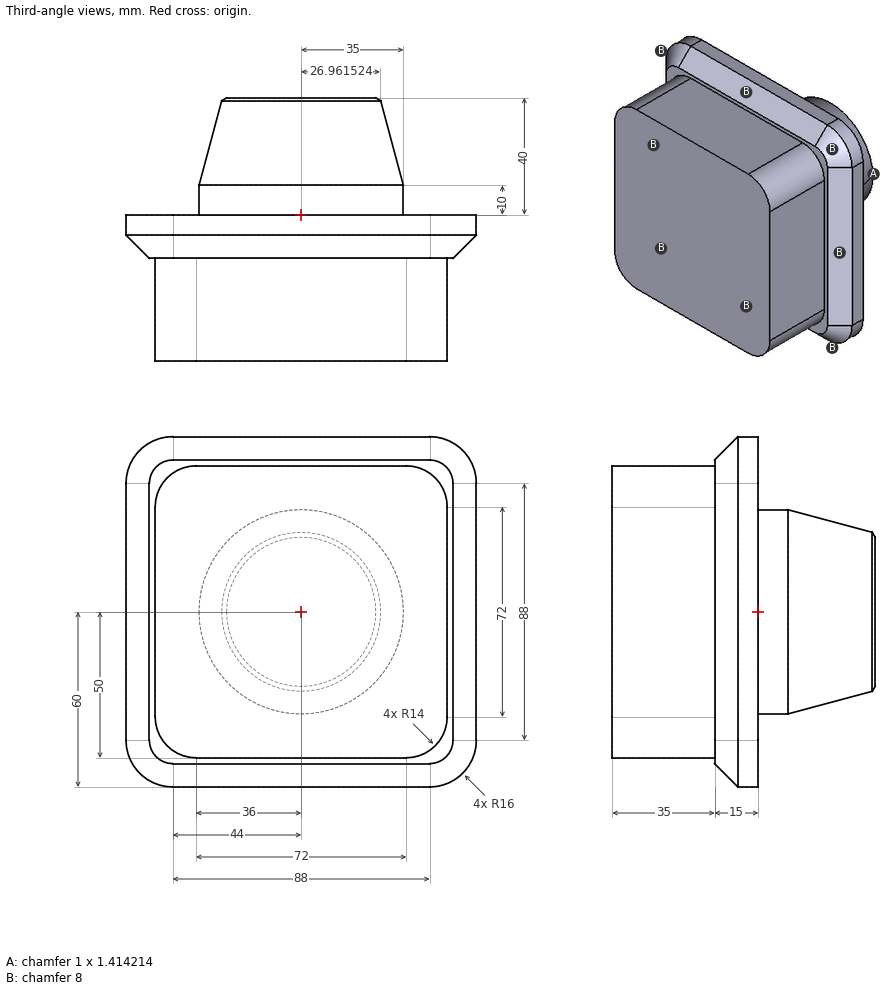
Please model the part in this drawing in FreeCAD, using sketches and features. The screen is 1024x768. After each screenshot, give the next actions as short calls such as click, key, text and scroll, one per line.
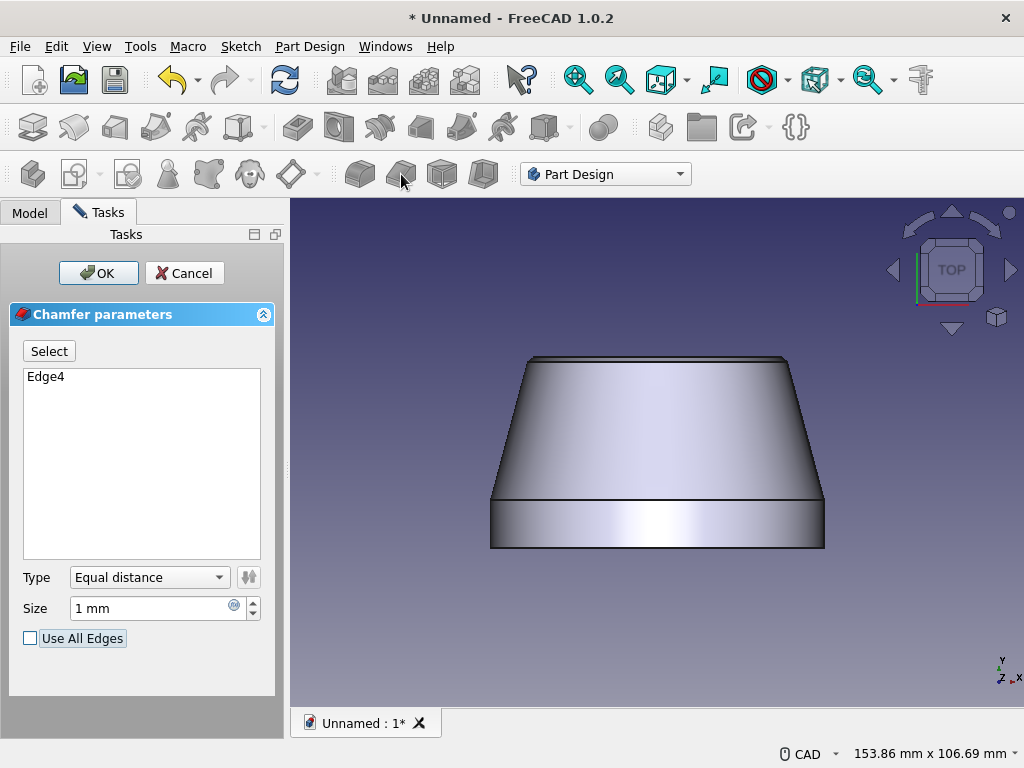
click(150, 578)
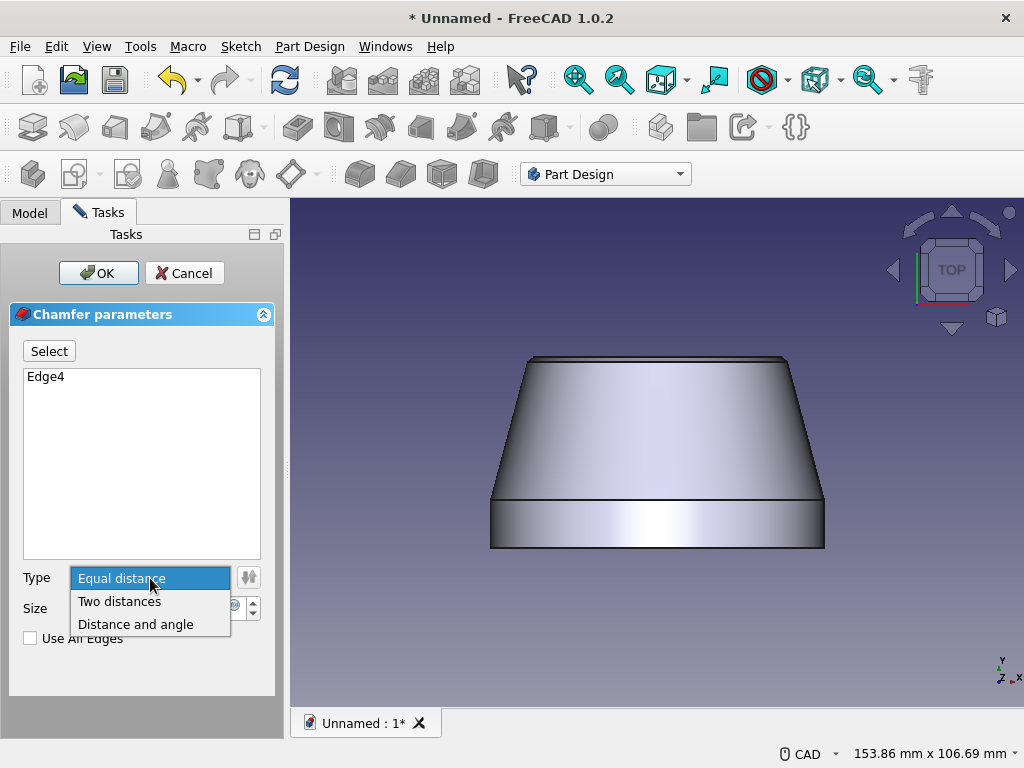
click(148, 602)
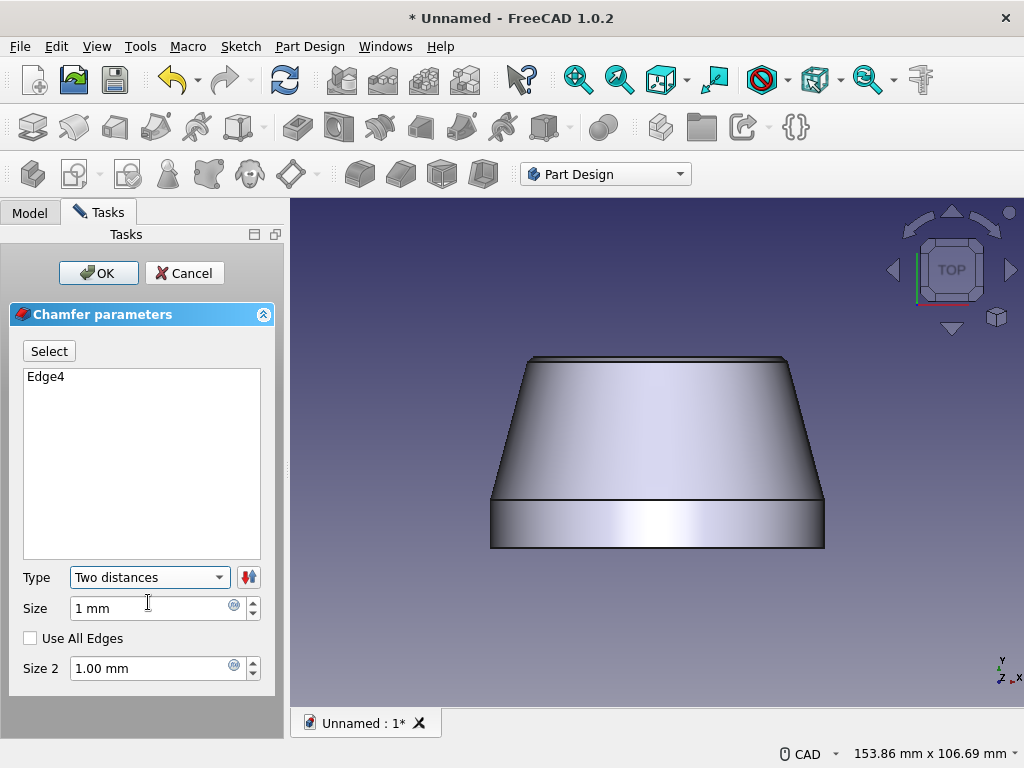
triple_click(158, 668)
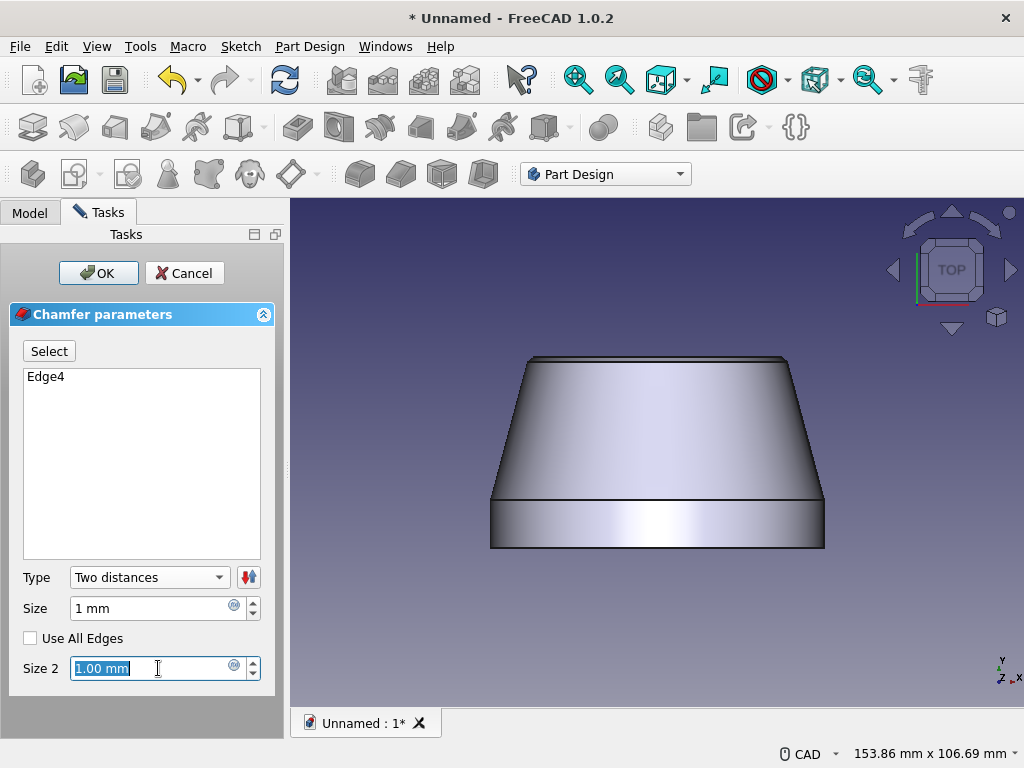
text(1.414214)
key(Tab)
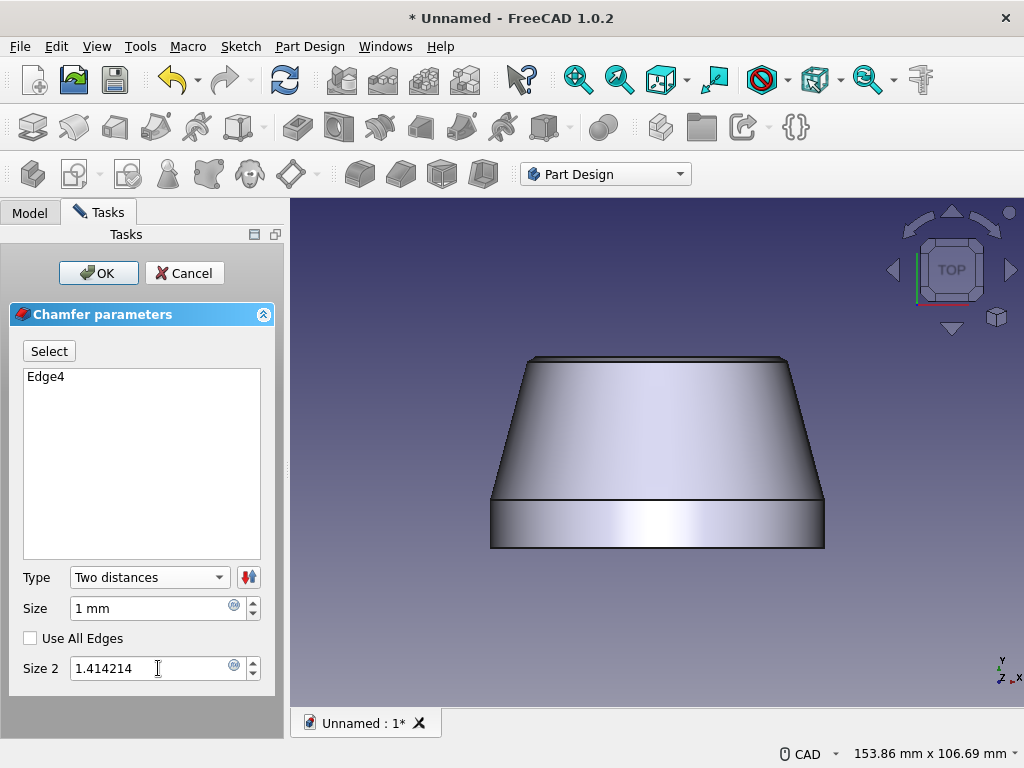
click(99, 273)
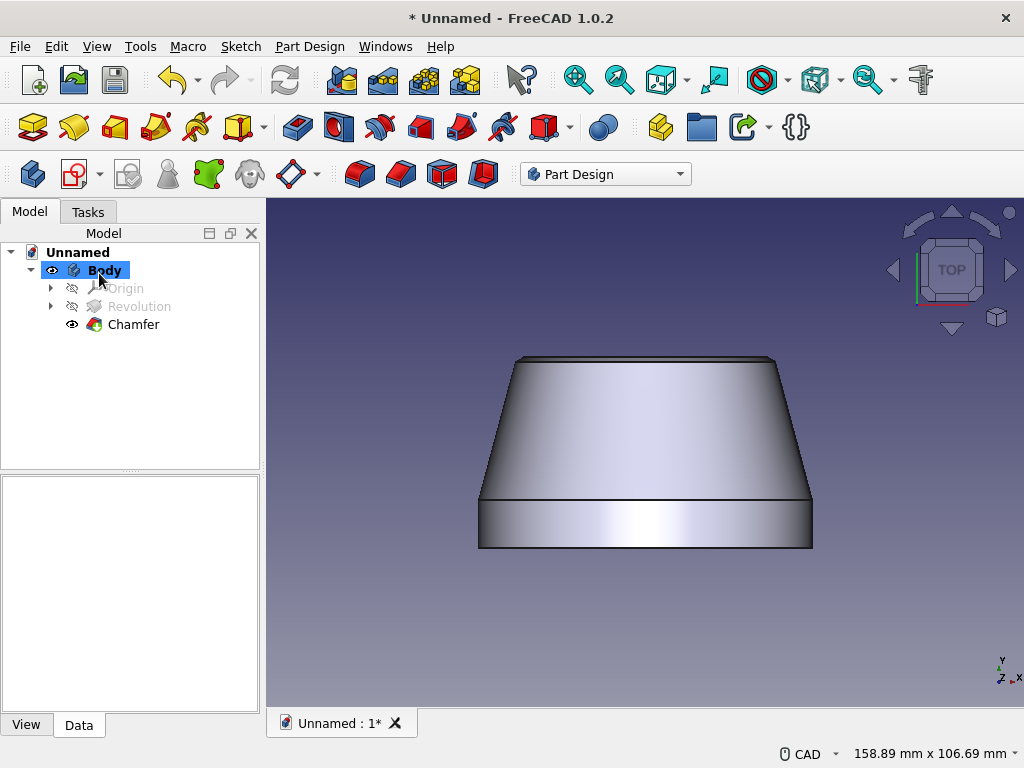
click(579, 80)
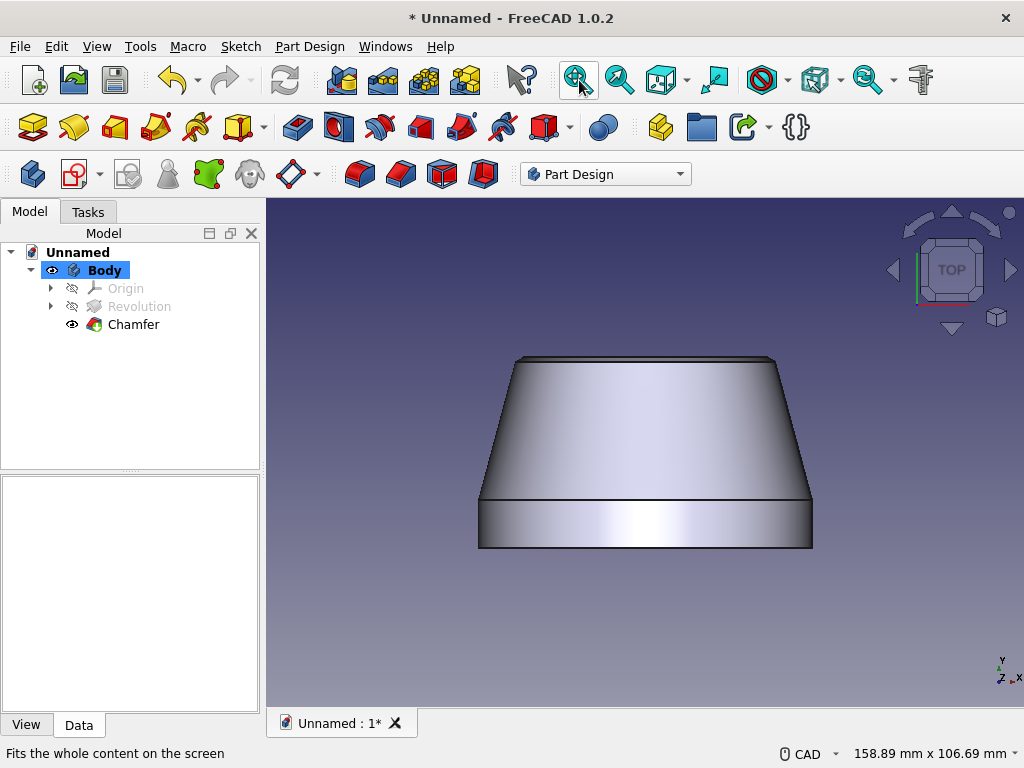
key(0)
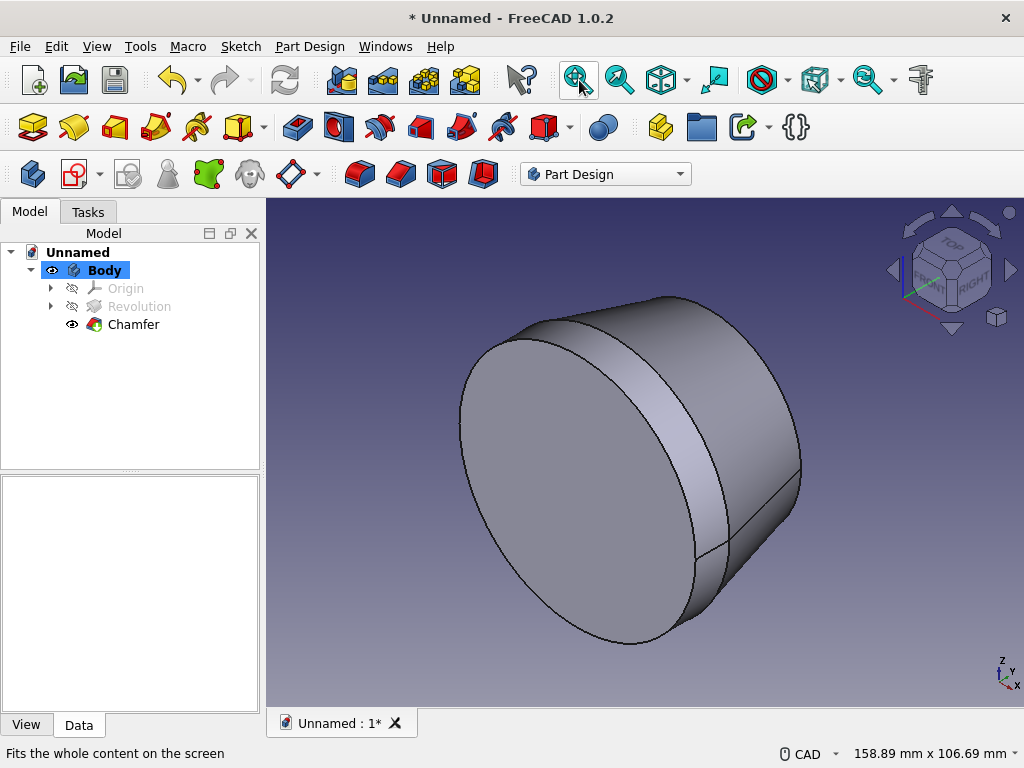
click(578, 490)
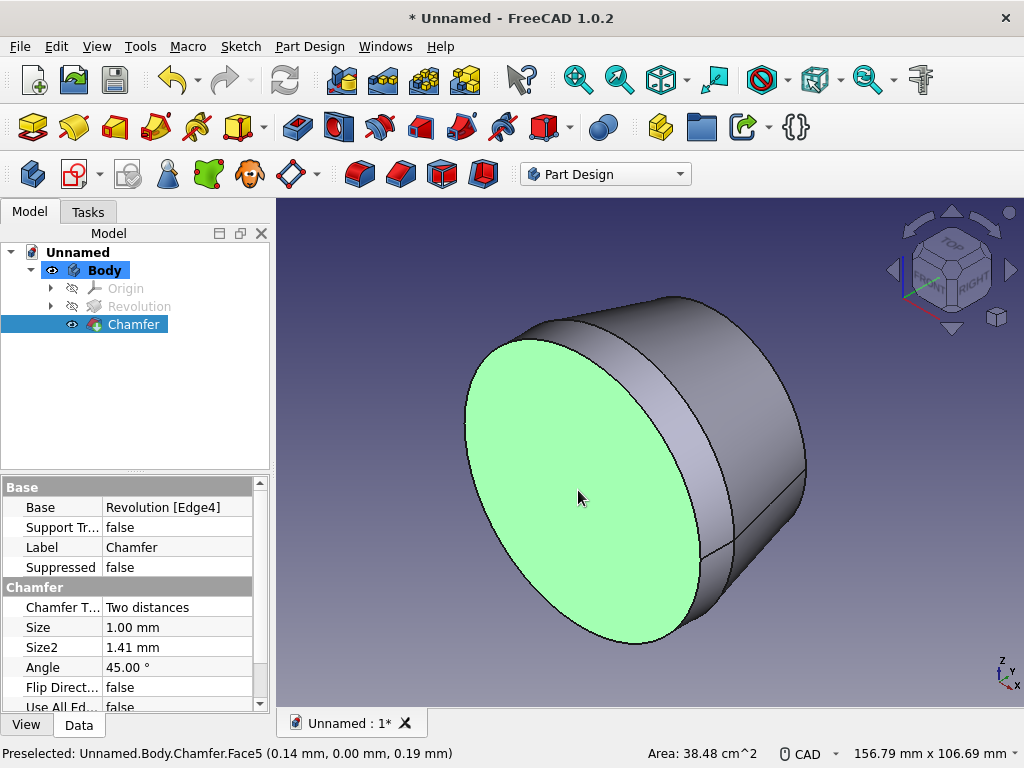
click(74, 174)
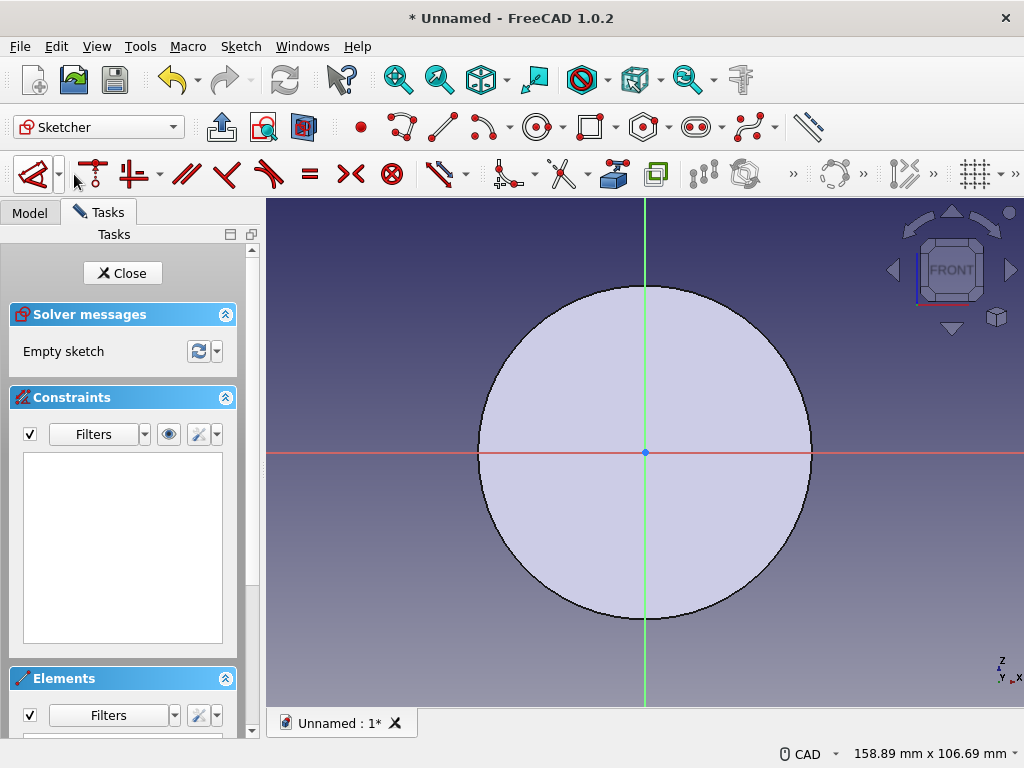
scroll(493, 452, down, 3)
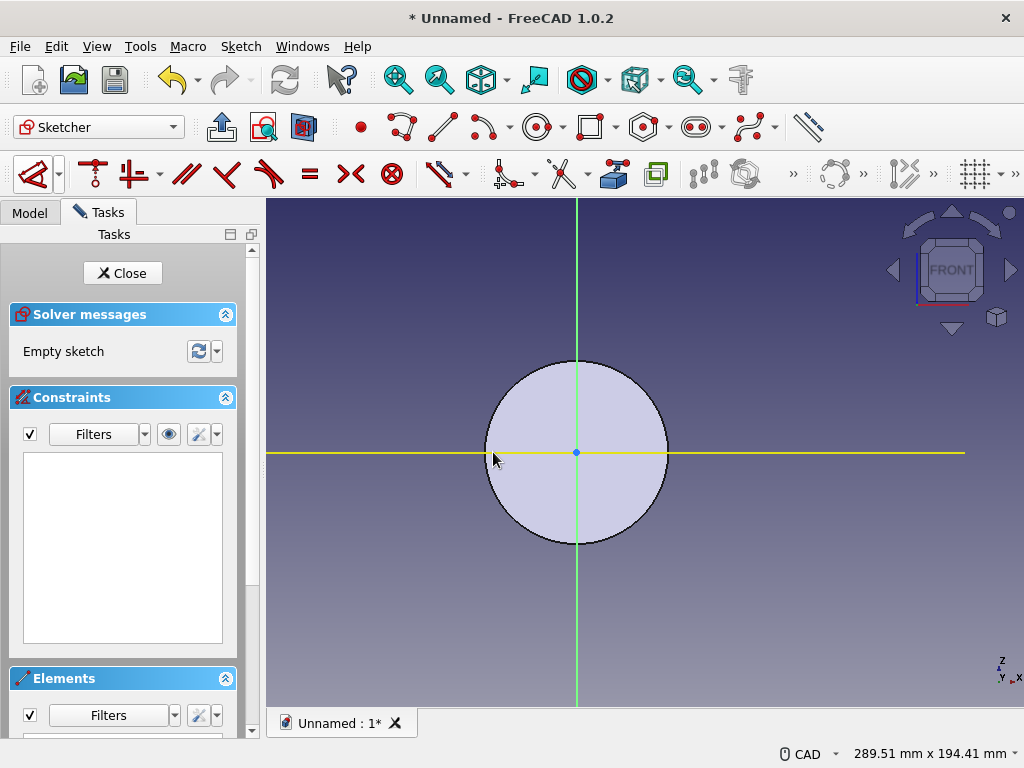
key(g)
key(l)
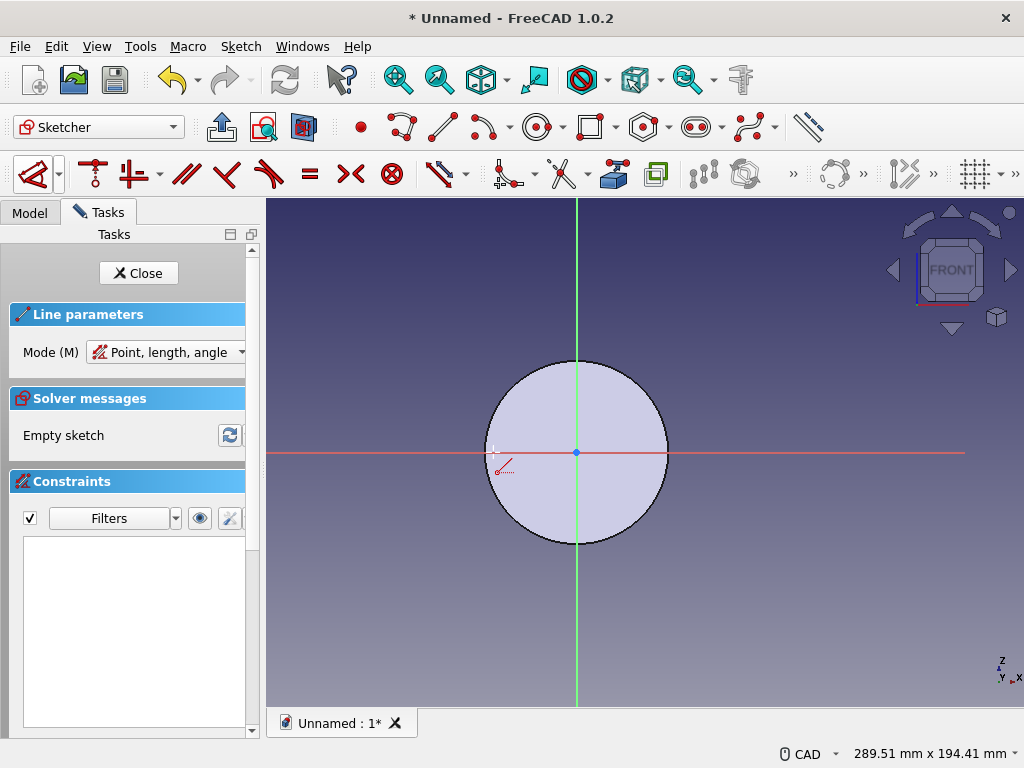
click(461, 610)
click(692, 610)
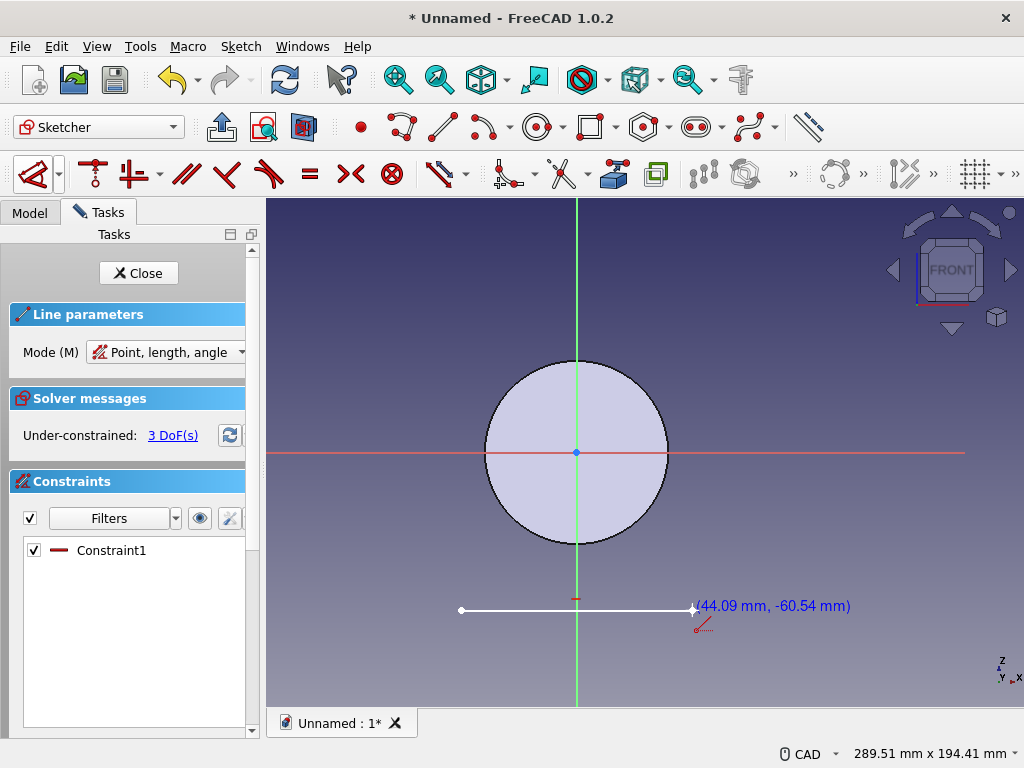
click(734, 568)
click(734, 337)